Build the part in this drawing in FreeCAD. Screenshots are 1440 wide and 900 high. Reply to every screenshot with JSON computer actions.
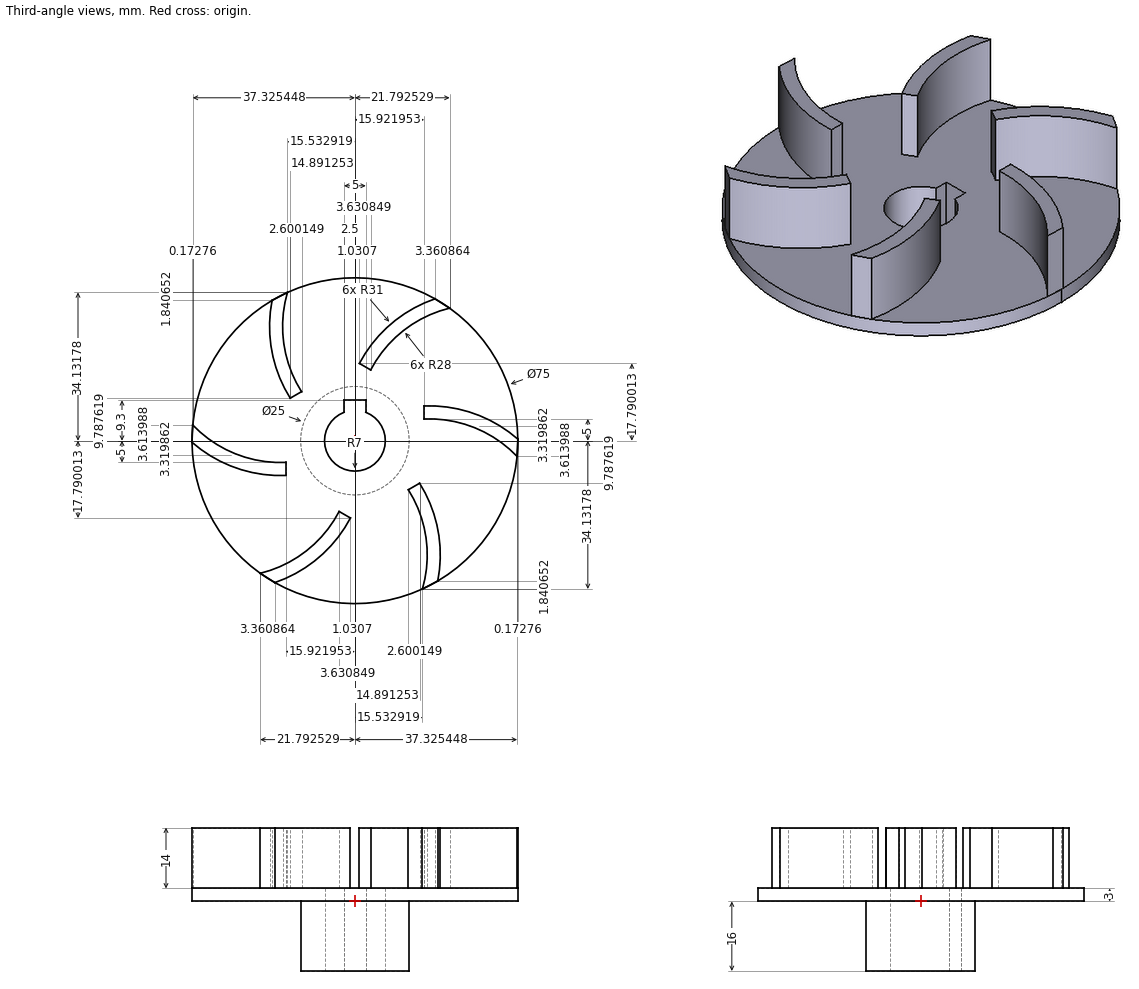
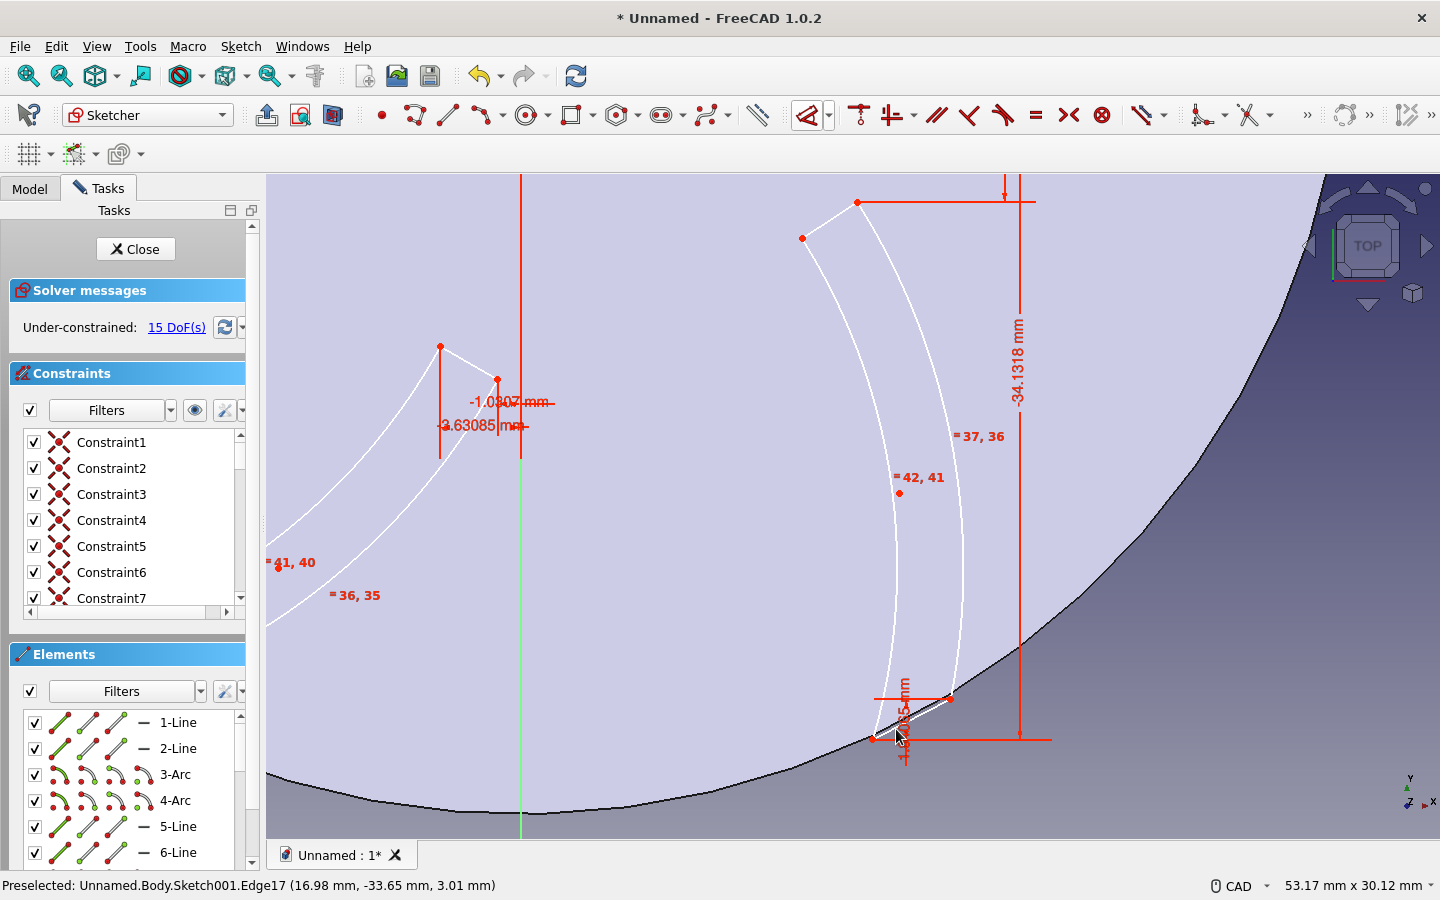
{"action": "left_click", "coordinate": [841, 213]}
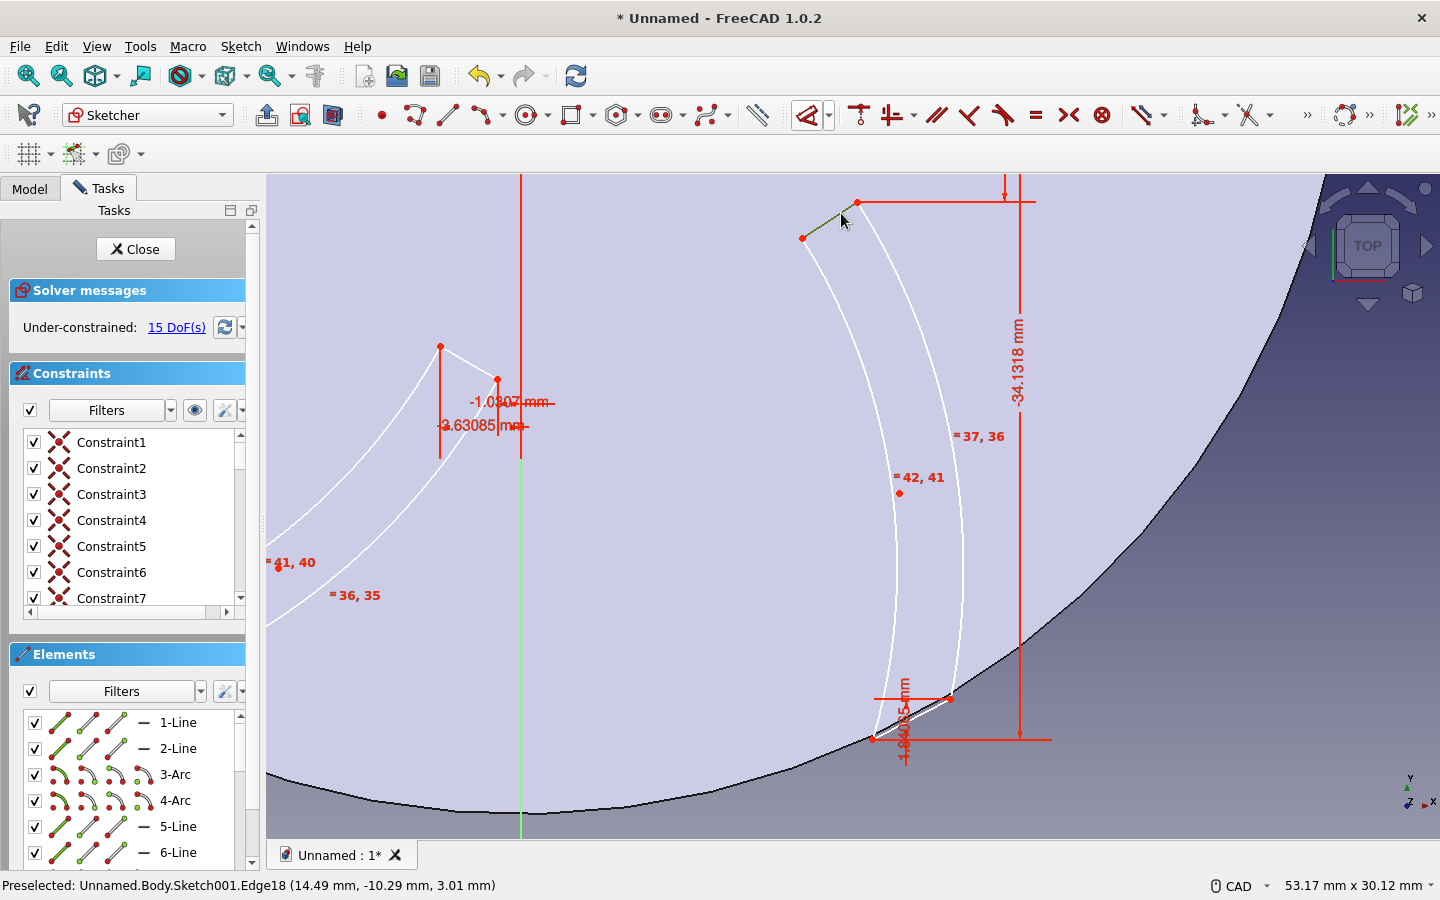
{"action": "key", "text": "l"}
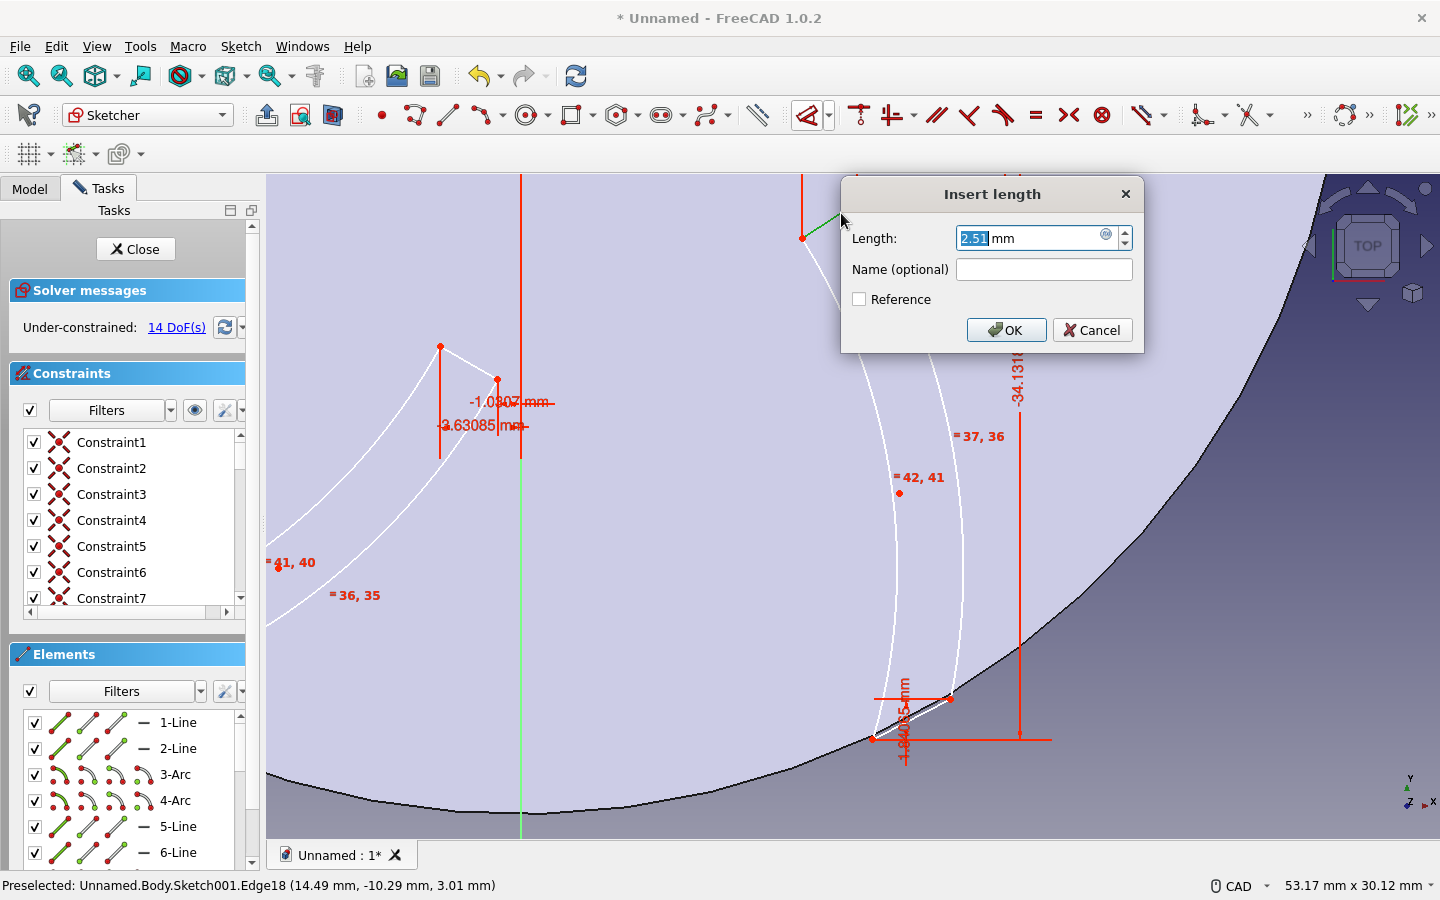
{"action": "type", "text": "2.600149"}
{"action": "key", "text": "Return"}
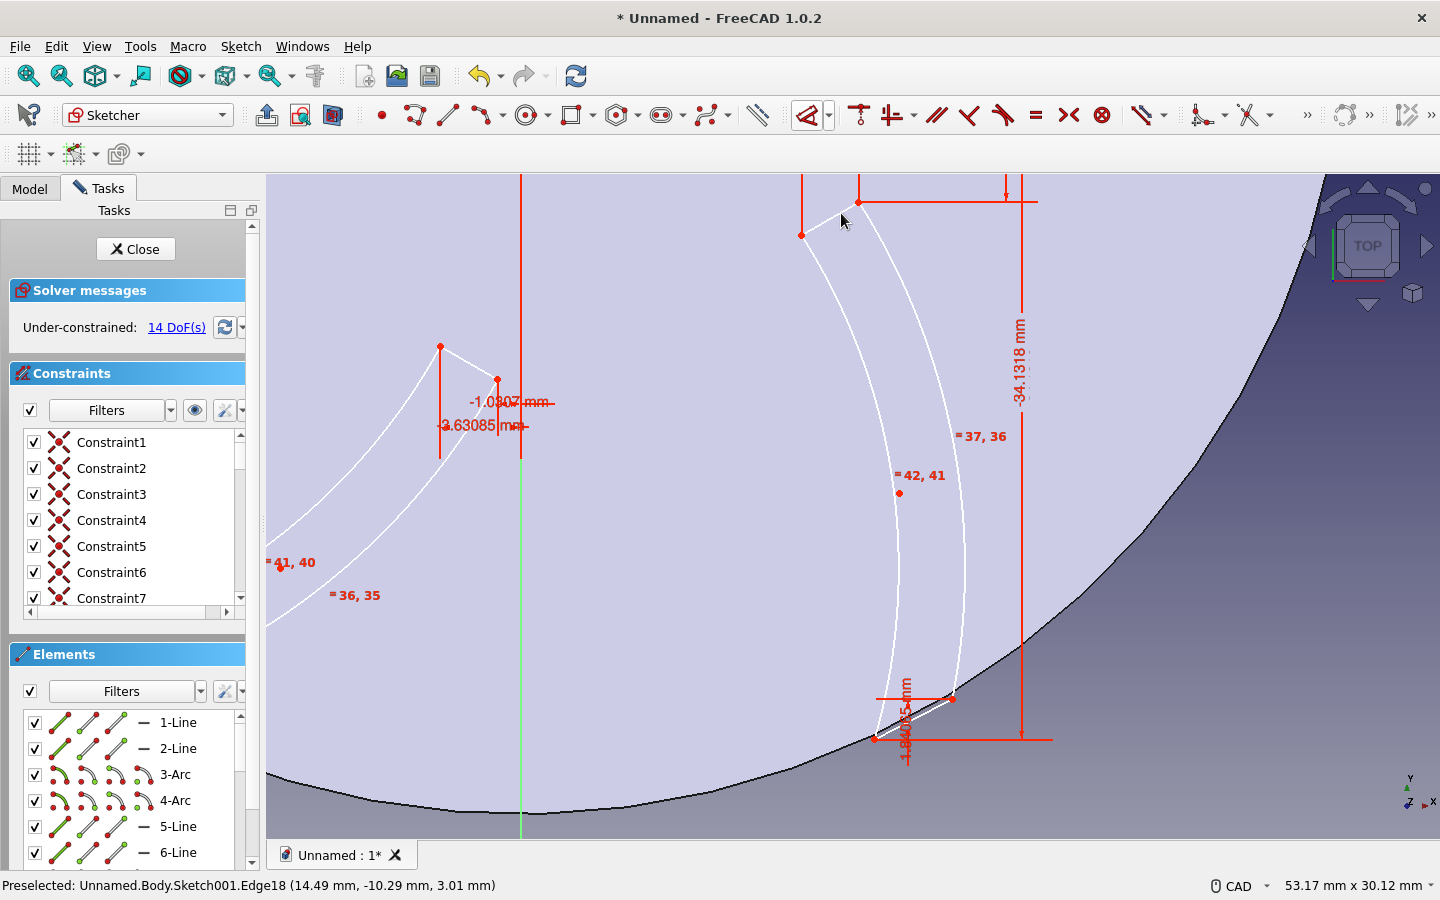
{"action": "scroll", "coordinate": [898, 731], "scroll_direction": "down", "scroll_amount": 6}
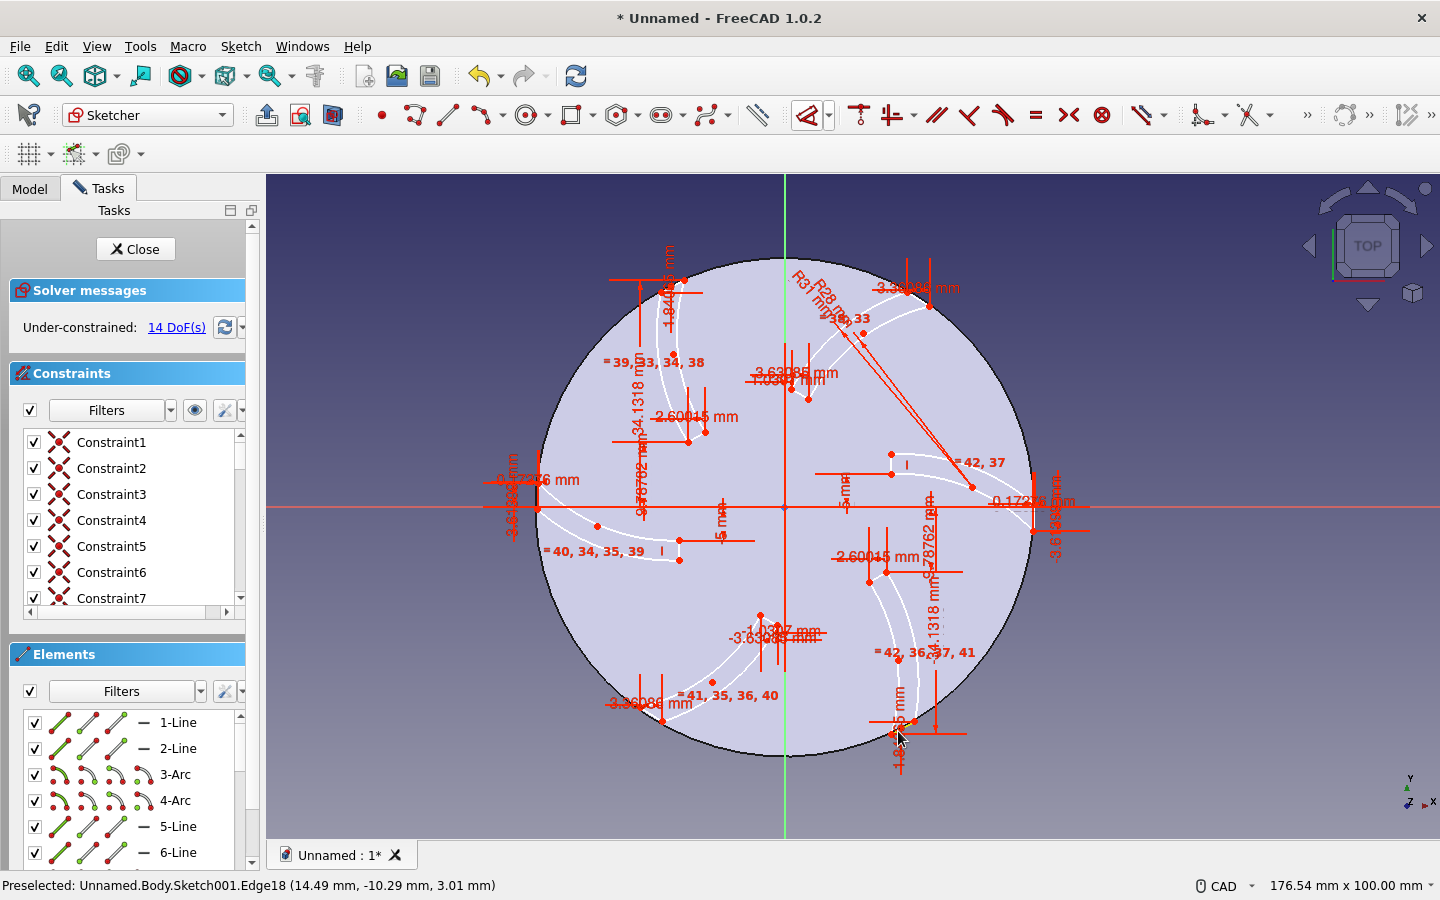
{"action": "scroll", "coordinate": [973, 488], "scroll_direction": "up", "scroll_amount": 3}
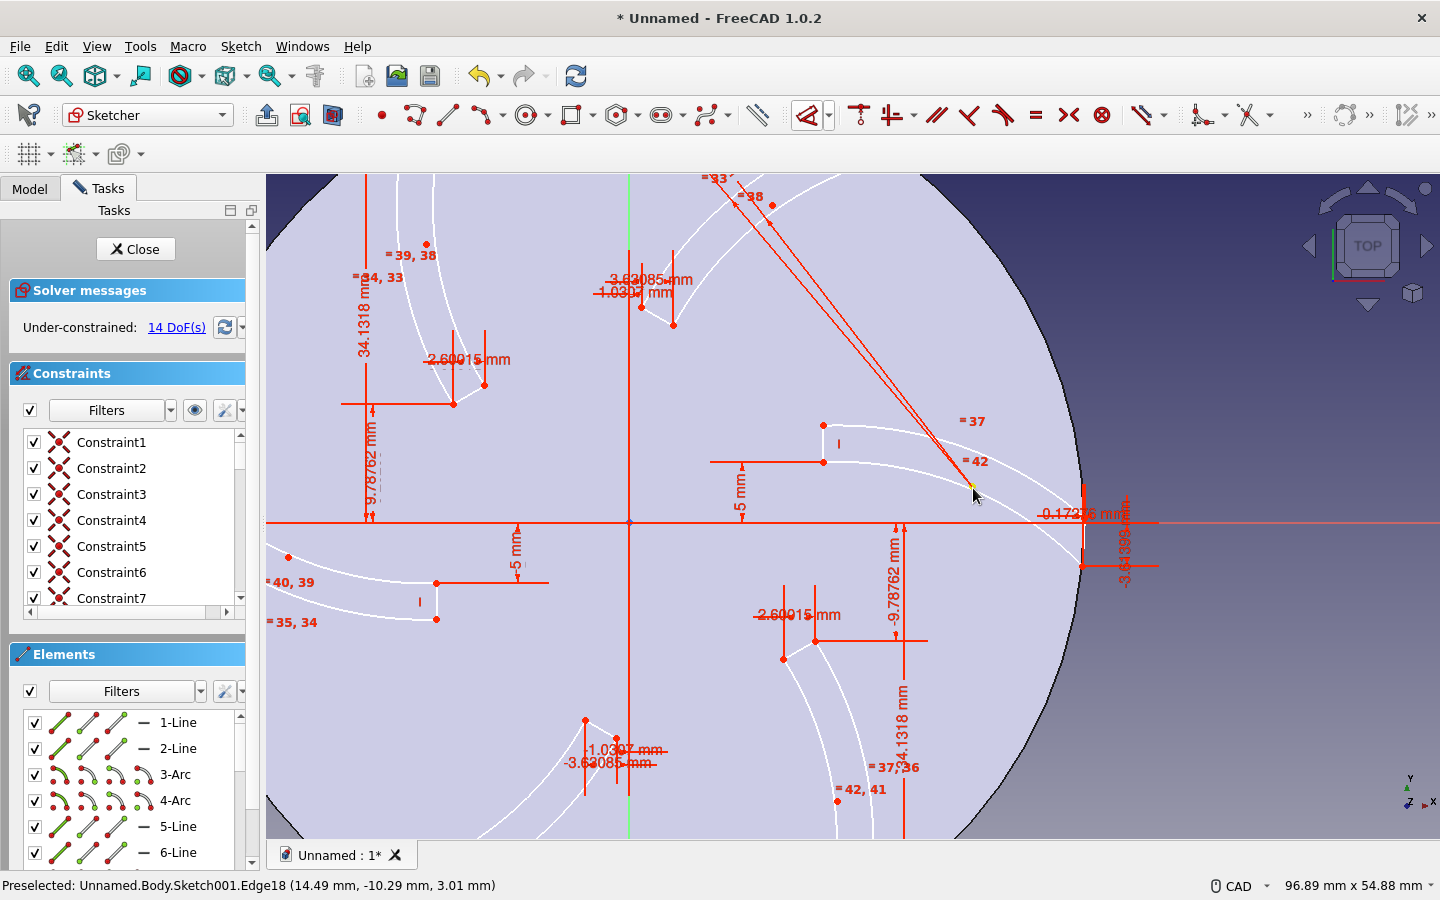
{"action": "left_click", "coordinate": [972, 487]}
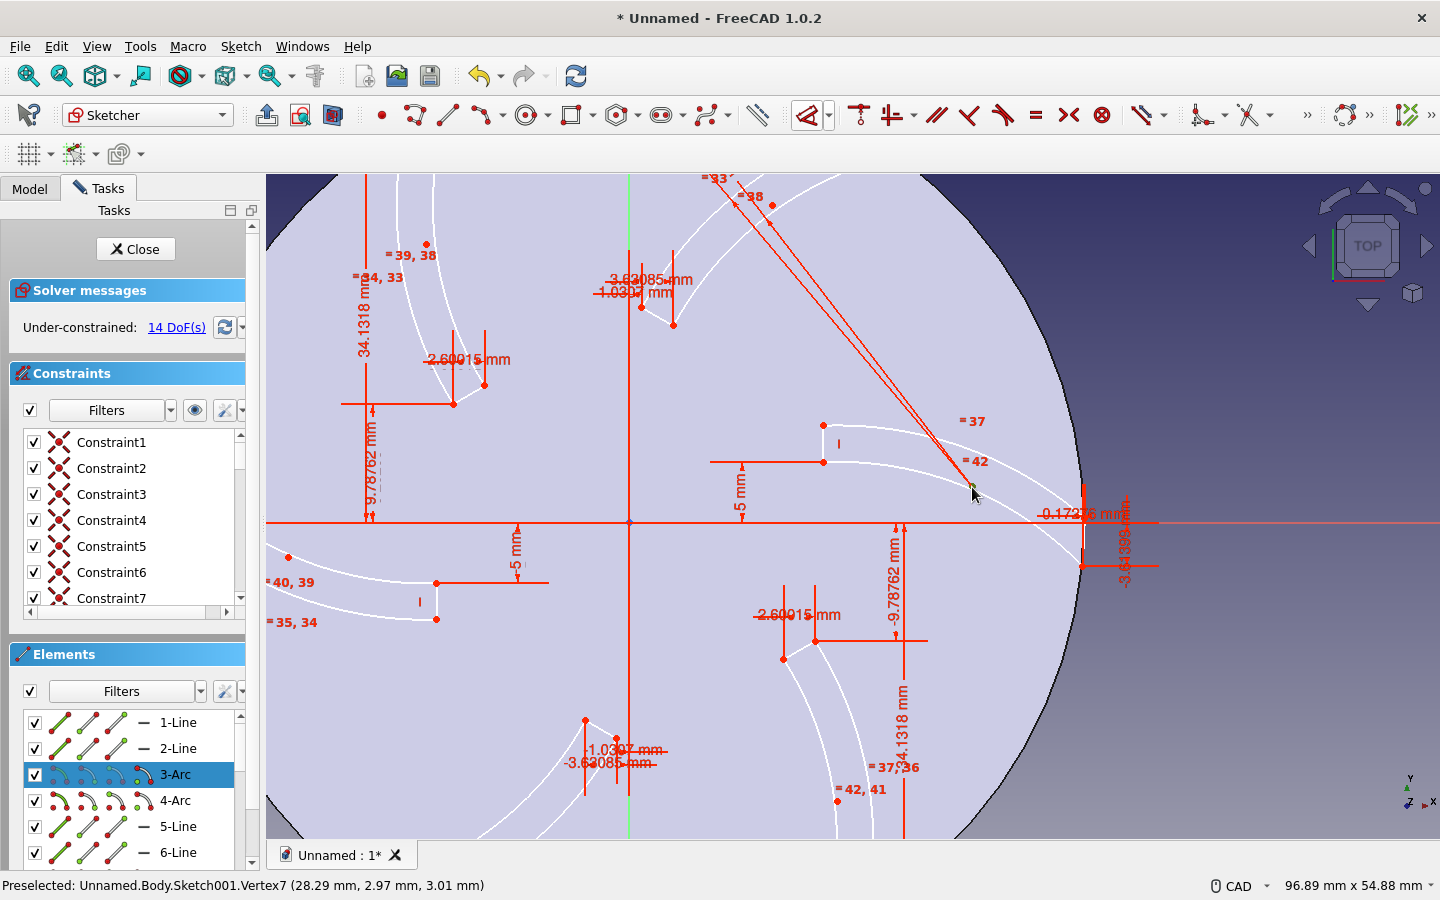
{"action": "key", "text": "i"}